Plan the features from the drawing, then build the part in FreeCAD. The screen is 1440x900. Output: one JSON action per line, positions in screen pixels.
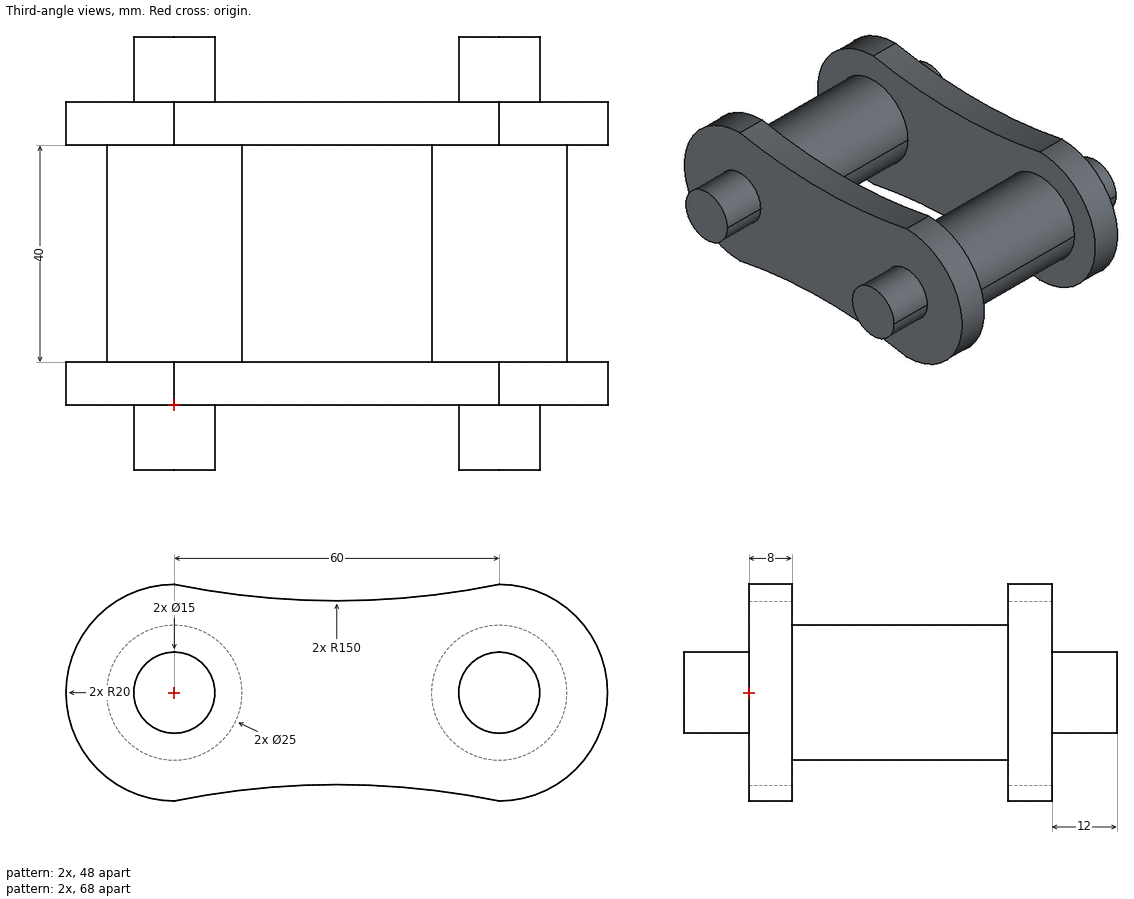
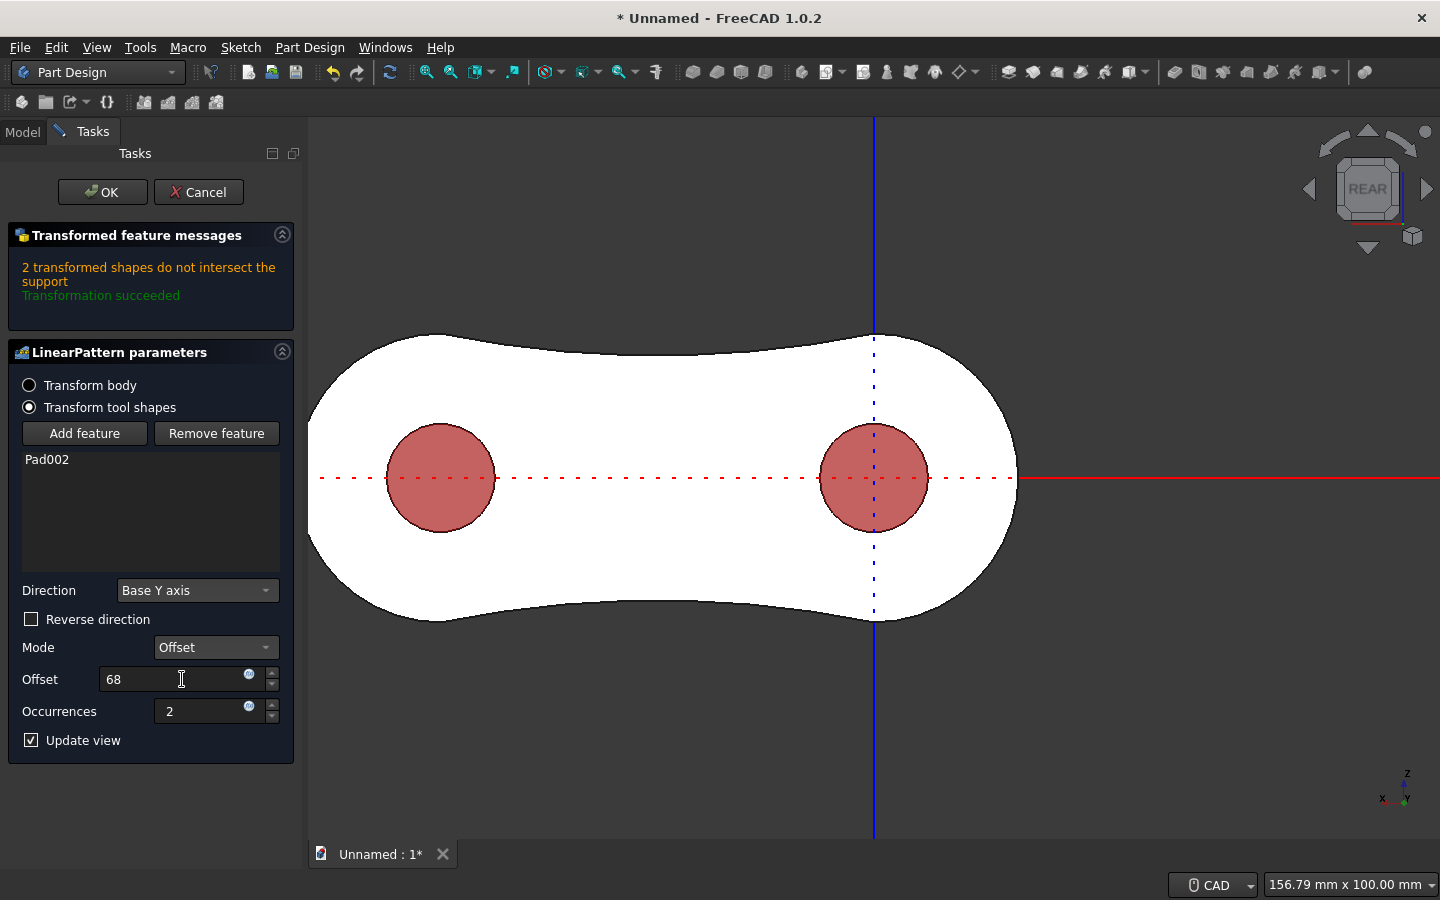
{"action": "triple_click", "coordinate": [209, 711]}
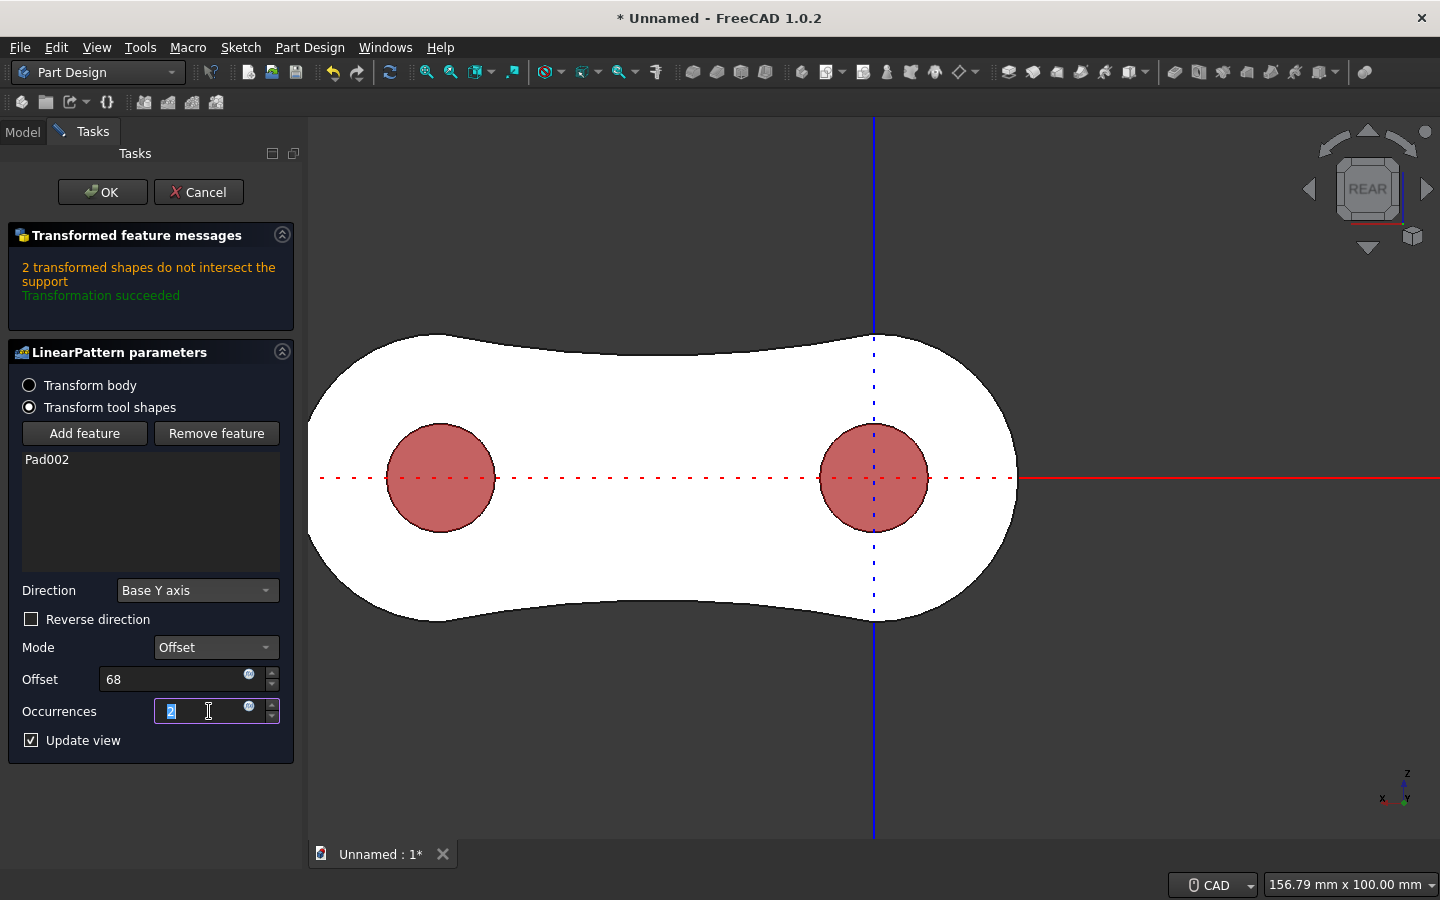
{"action": "type", "text": "2"}
{"action": "key", "text": "Tab"}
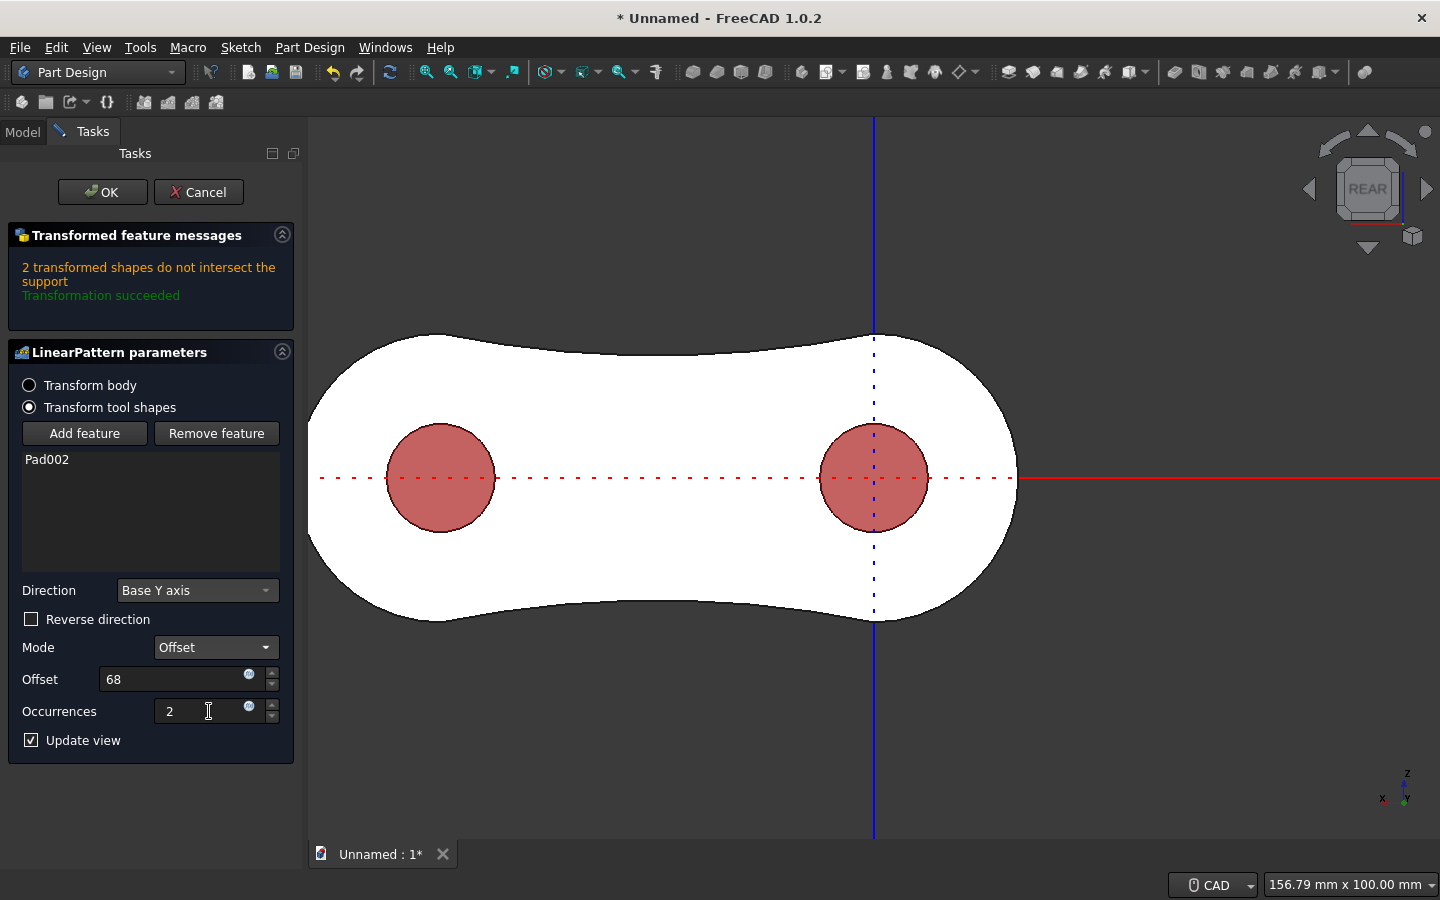
{"action": "left_click", "coordinate": [30, 619]}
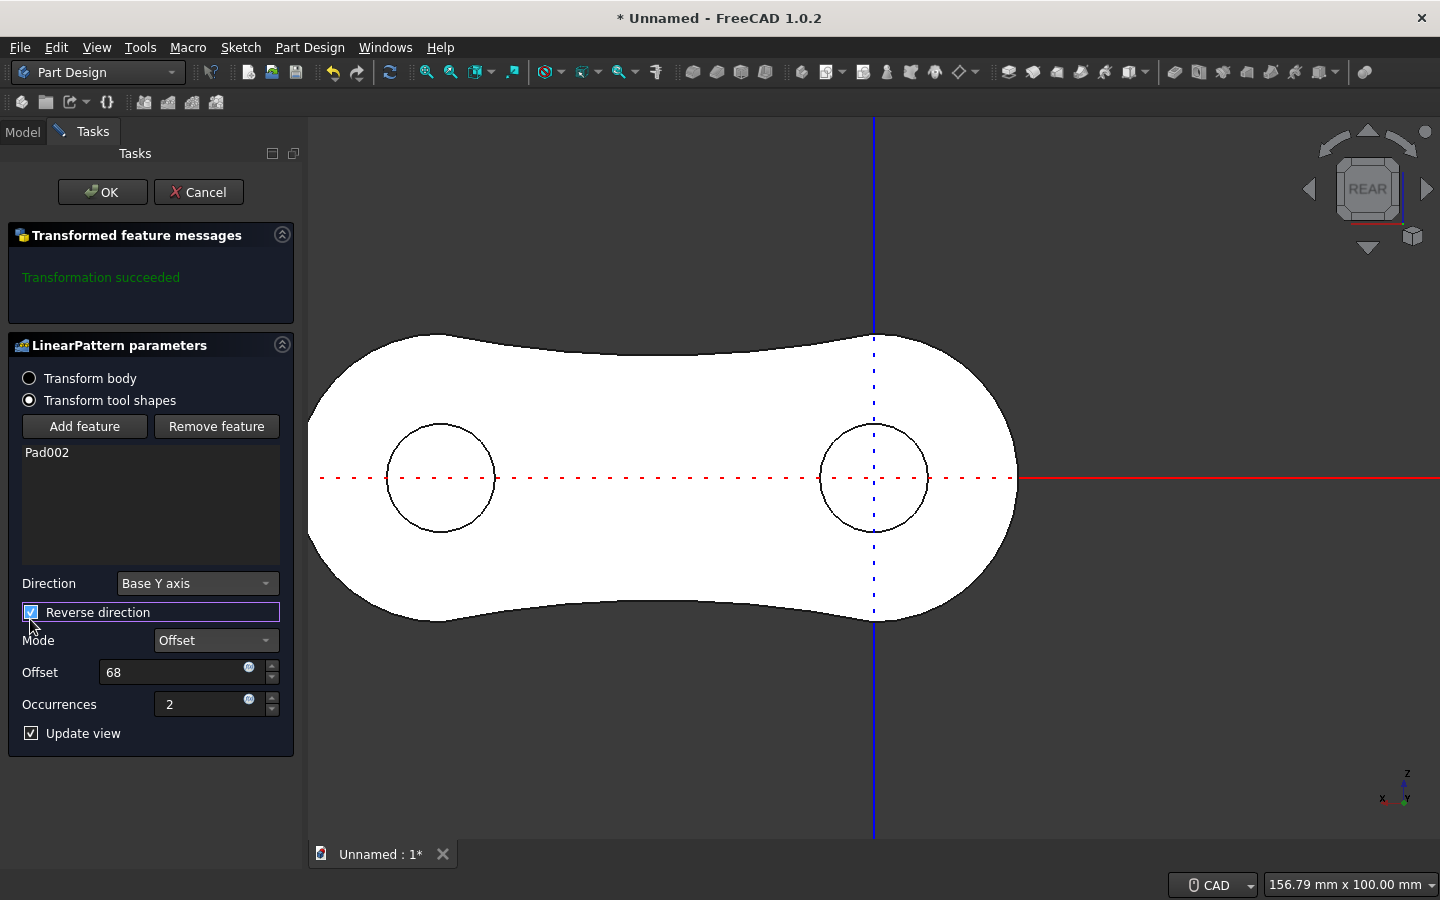
{"action": "left_click", "coordinate": [103, 192]}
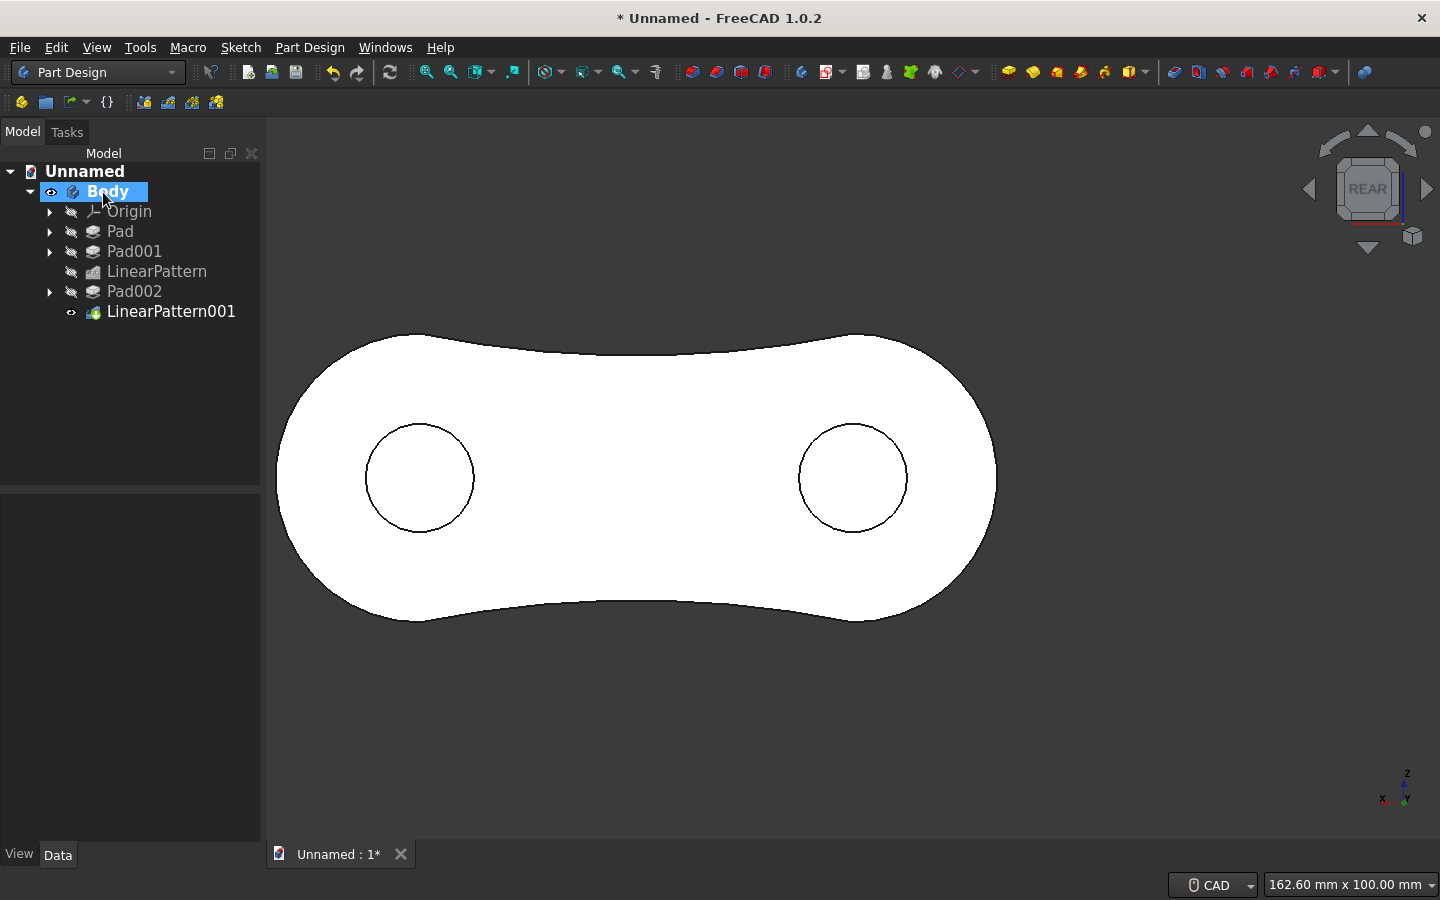
{"action": "key", "text": "0"}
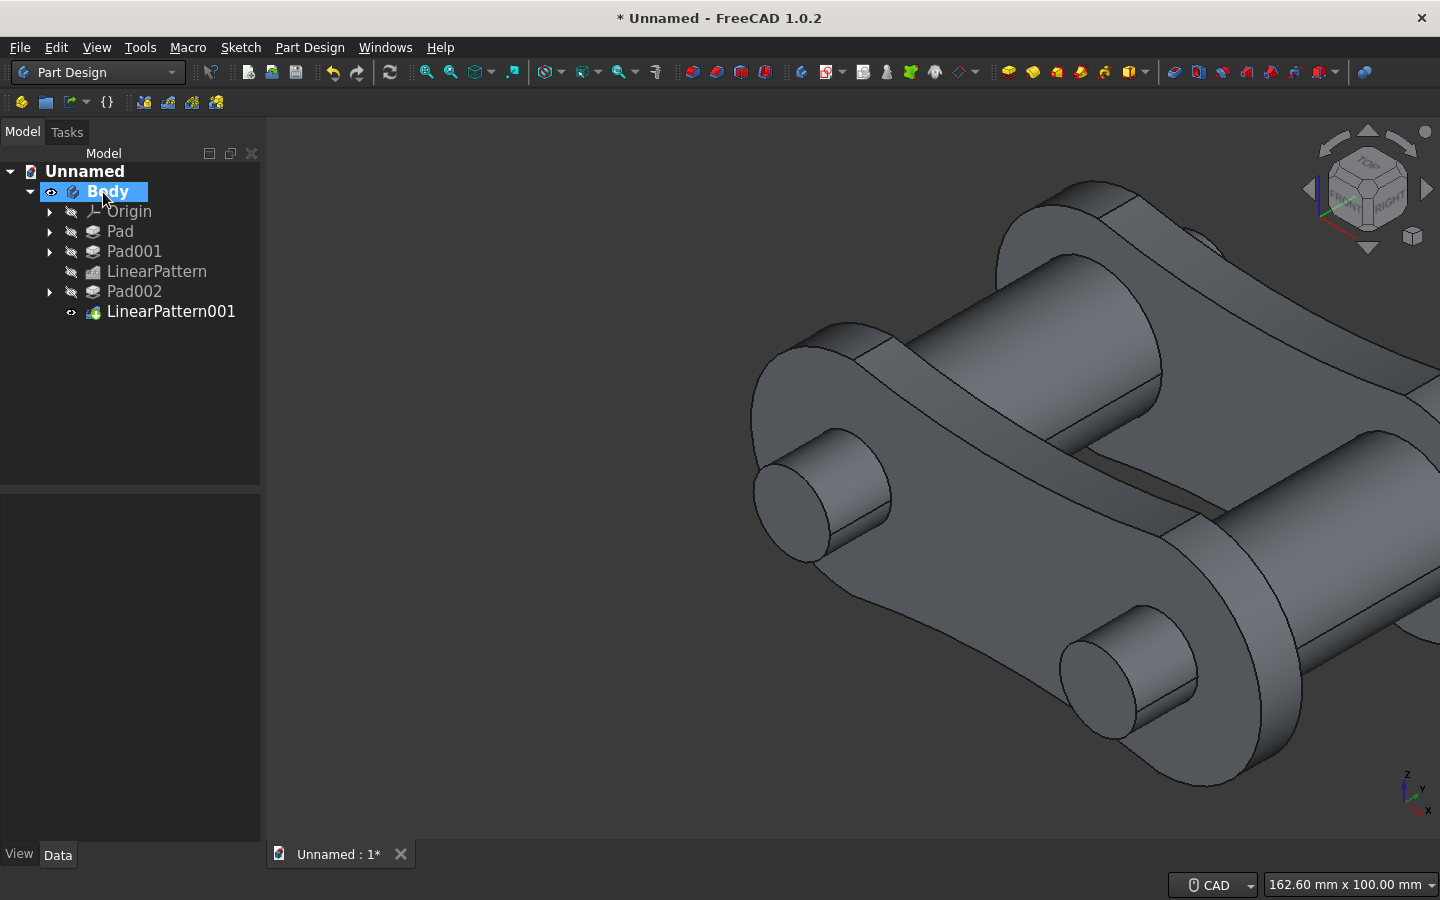
{"action": "left_click", "coordinate": [428, 72]}